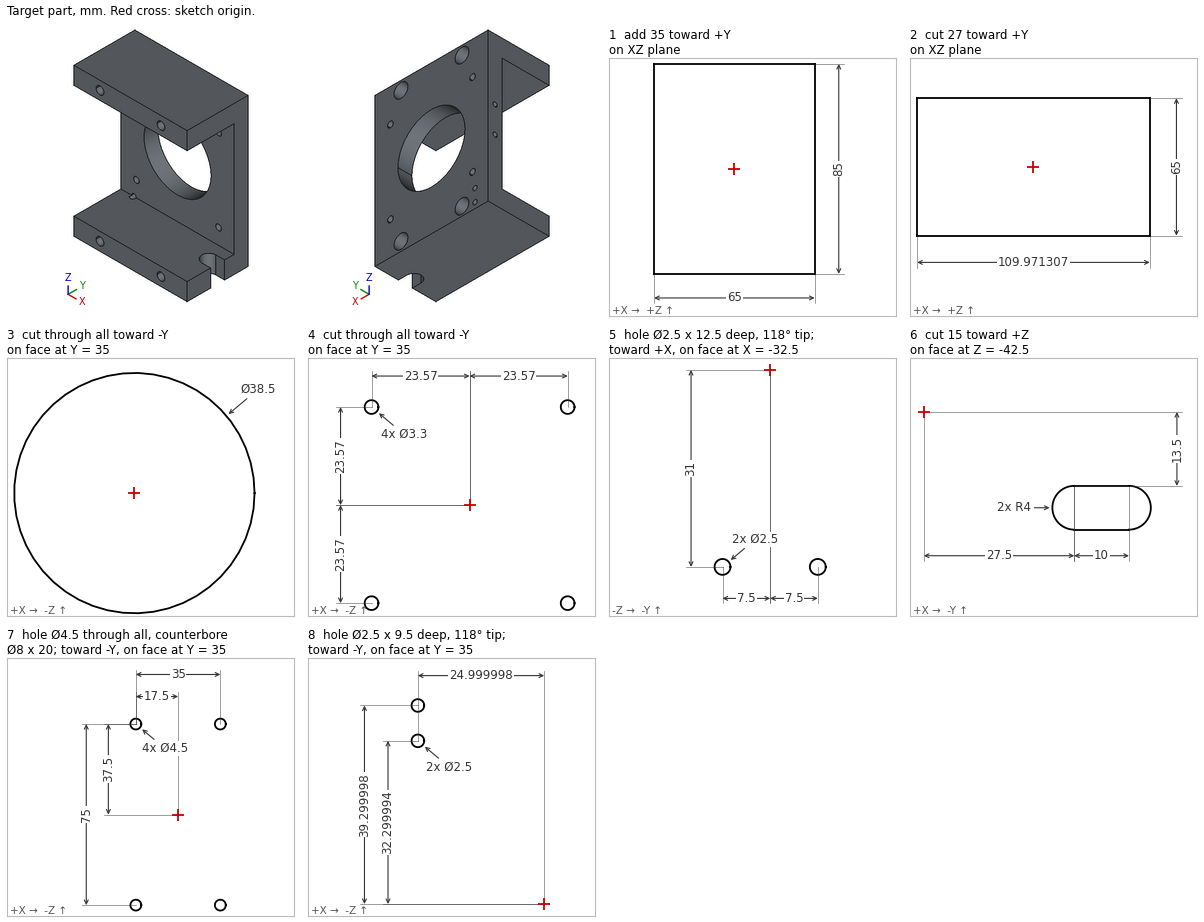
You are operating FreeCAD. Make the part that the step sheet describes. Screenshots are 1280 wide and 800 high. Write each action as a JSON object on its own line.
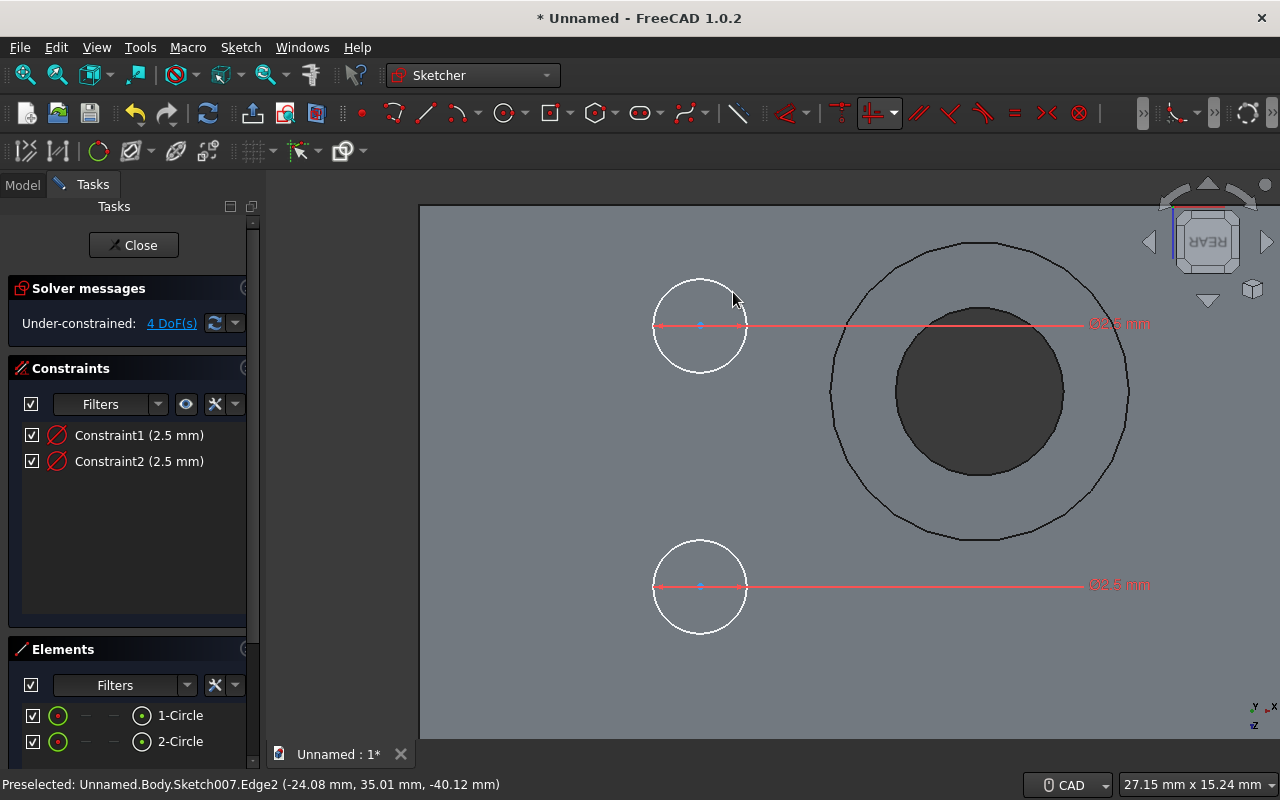
{"action": "left_click", "coordinate": [700, 587]}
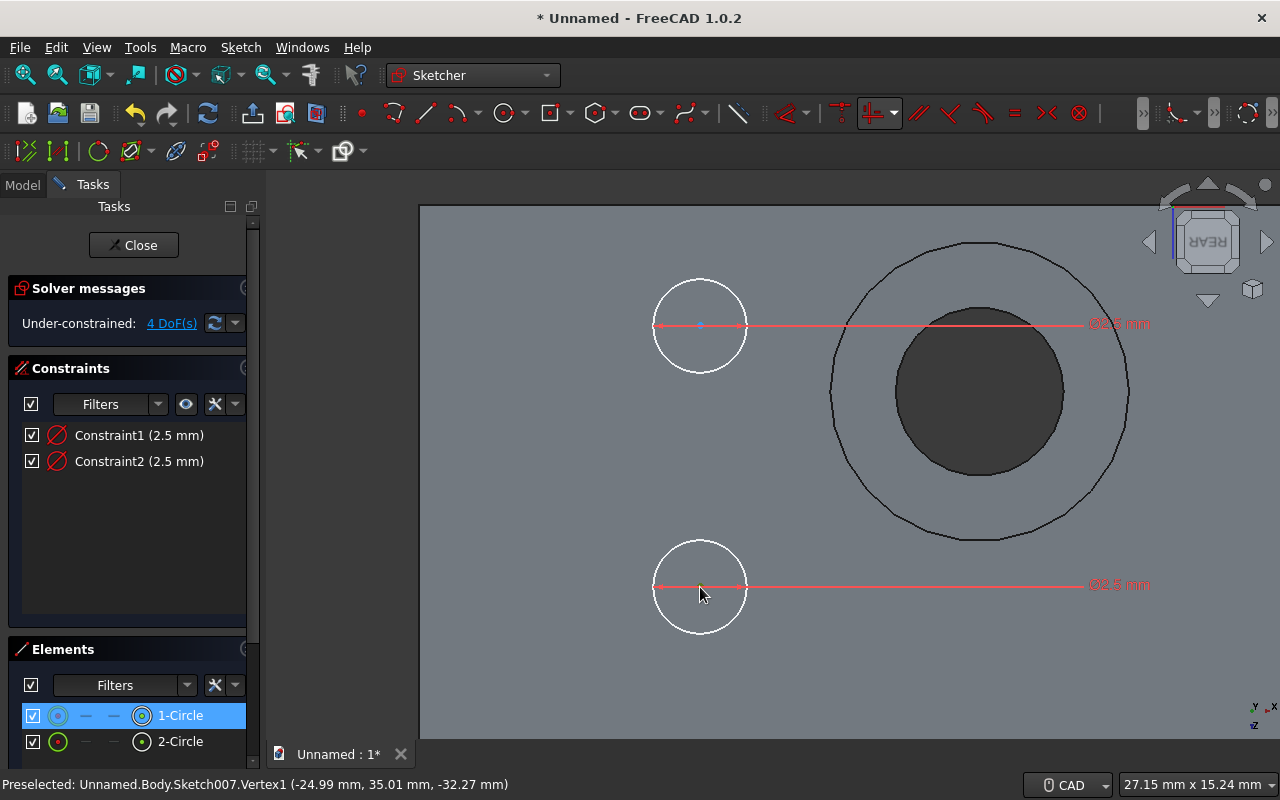
{"action": "left_click", "coordinate": [700, 326]}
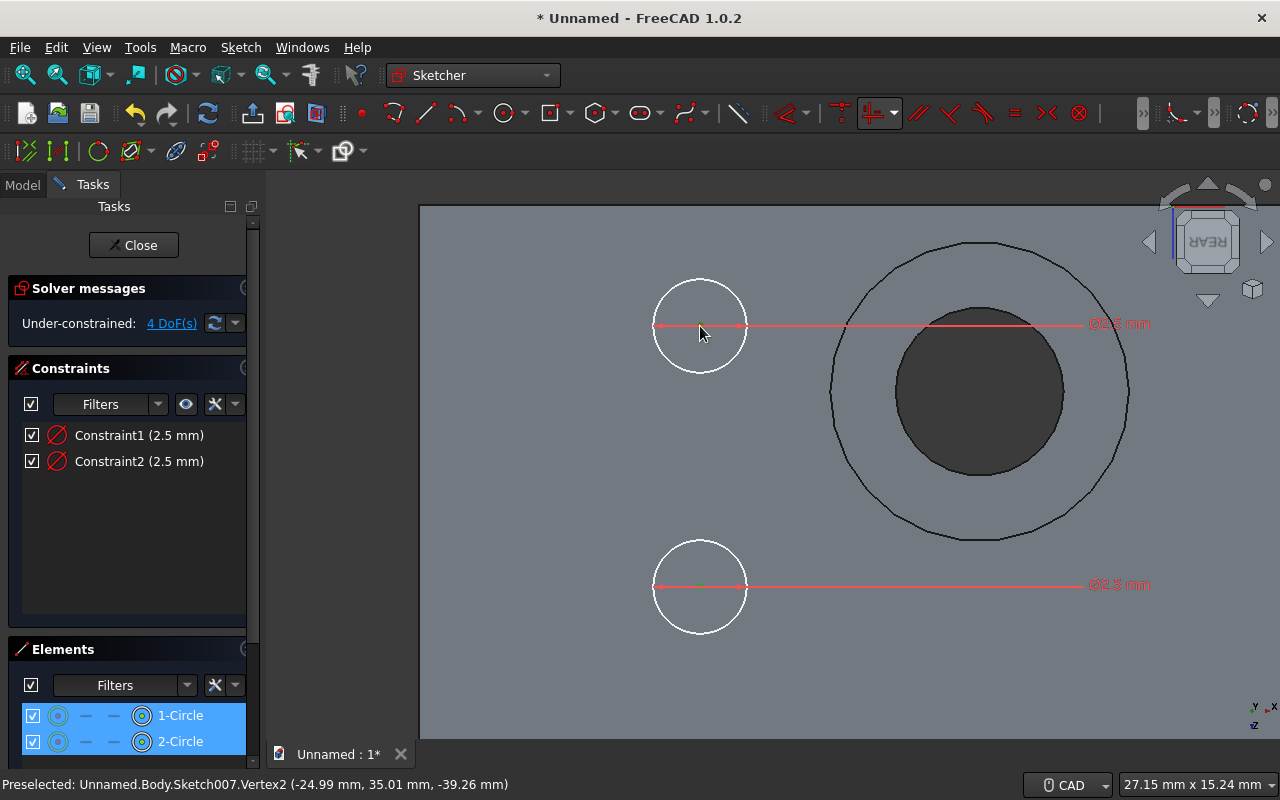
{"action": "key", "text": "v"}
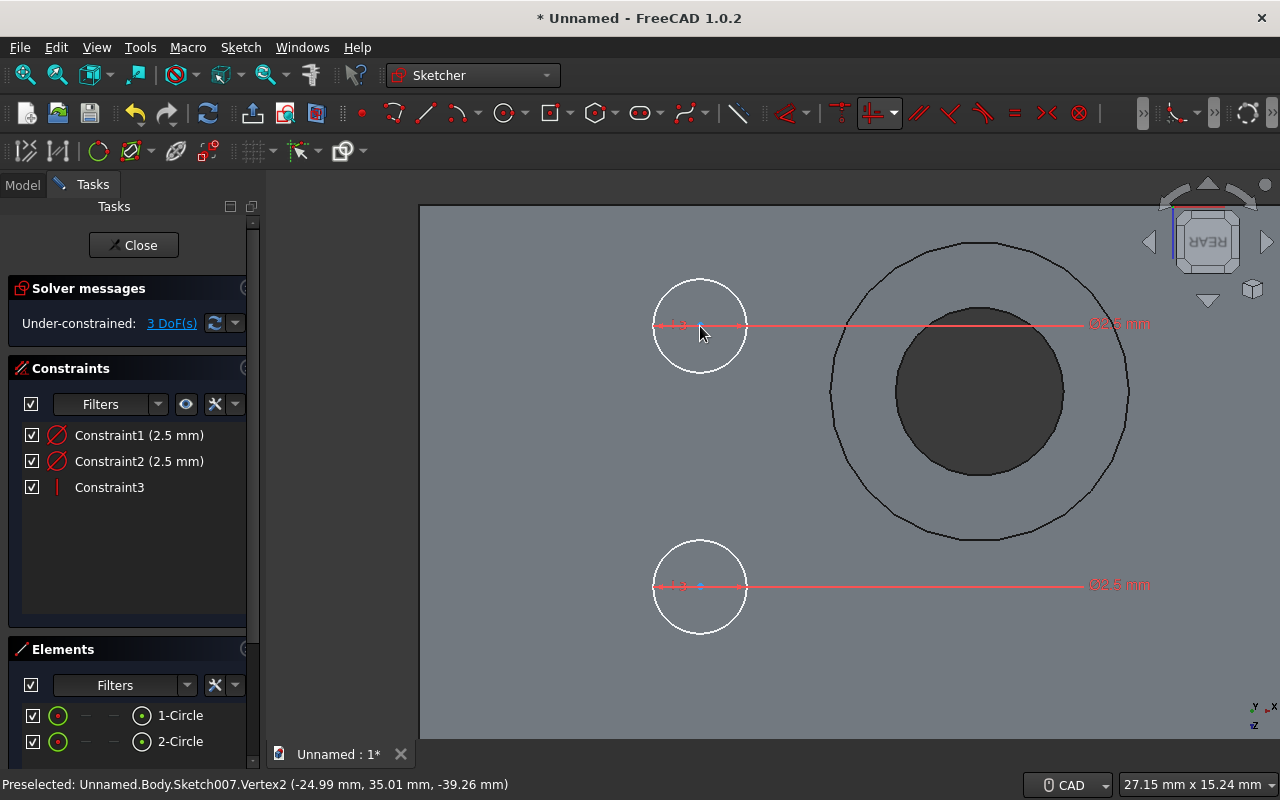
{"action": "left_click", "coordinate": [786, 114]}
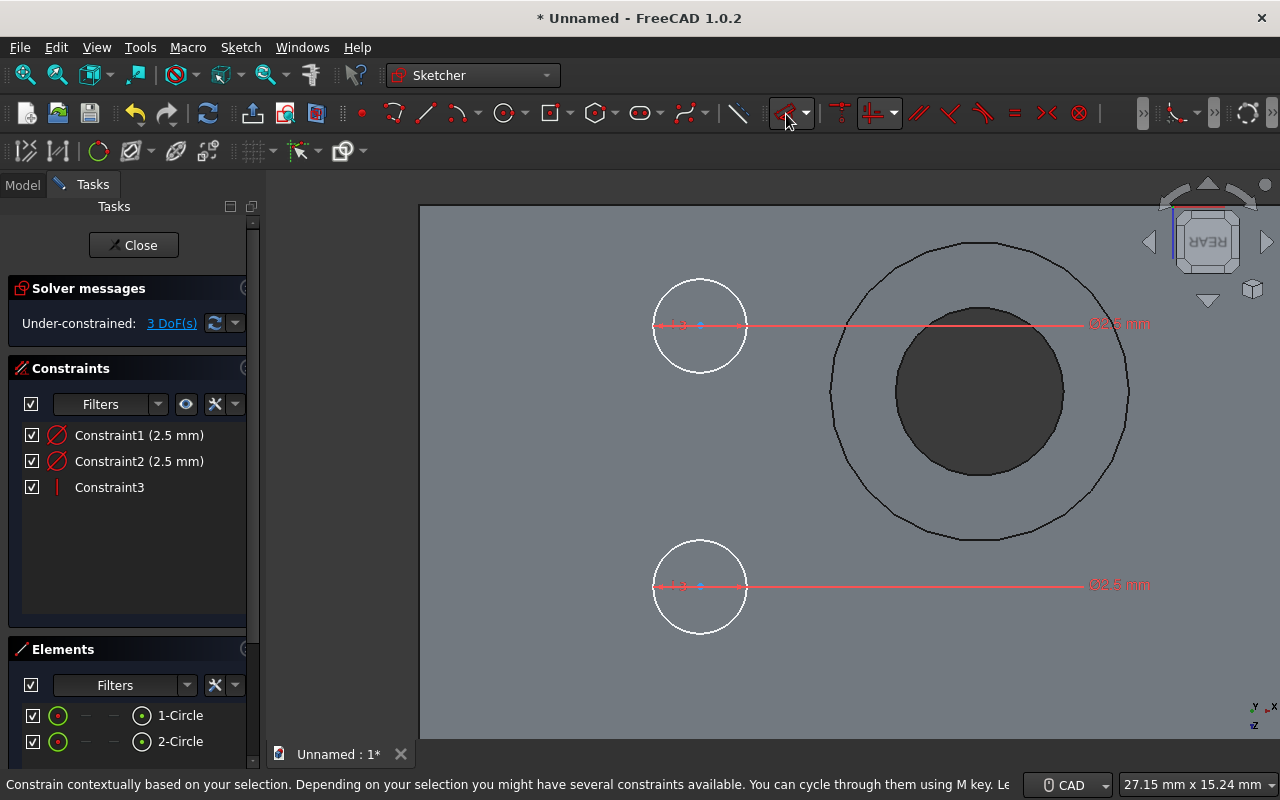
{"action": "left_click", "coordinate": [700, 587]}
{"action": "left_click", "coordinate": [908, 553]}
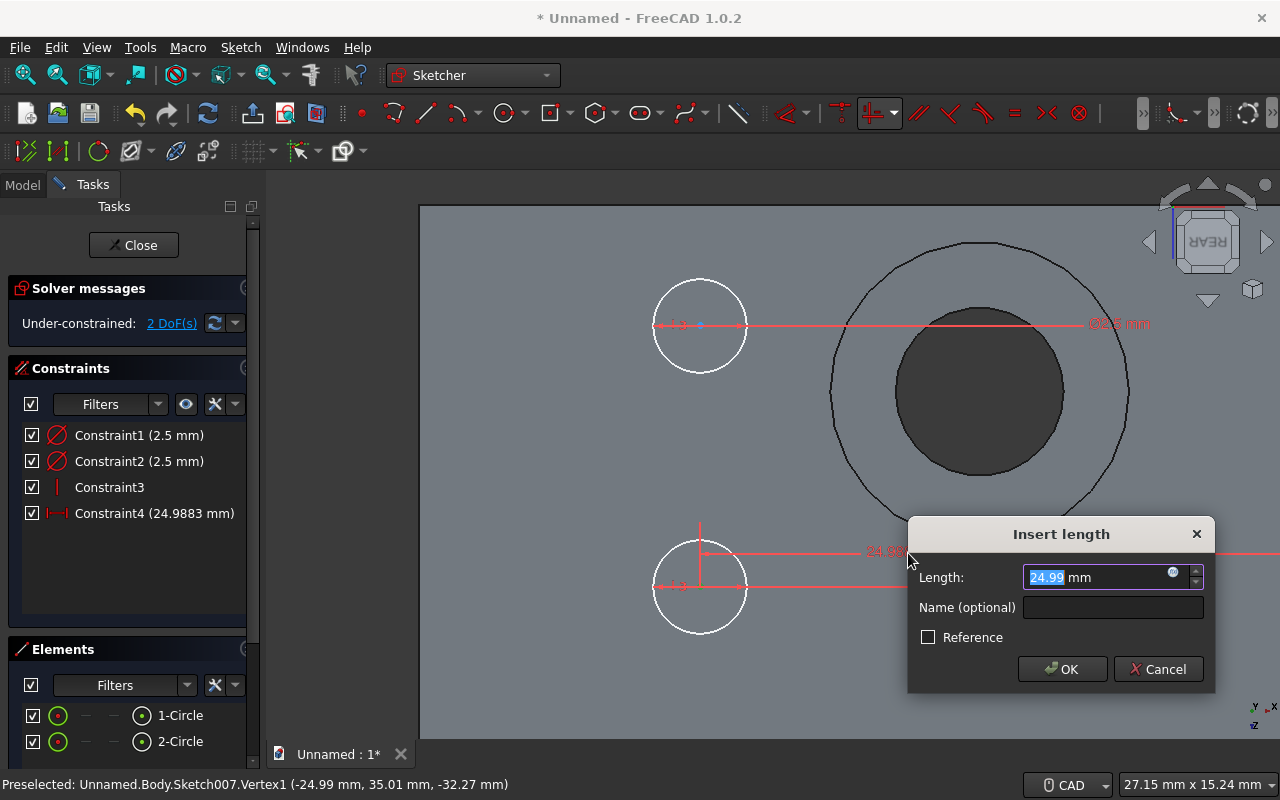
{"action": "type", "text": "24.999998"}
{"action": "key", "text": "Return"}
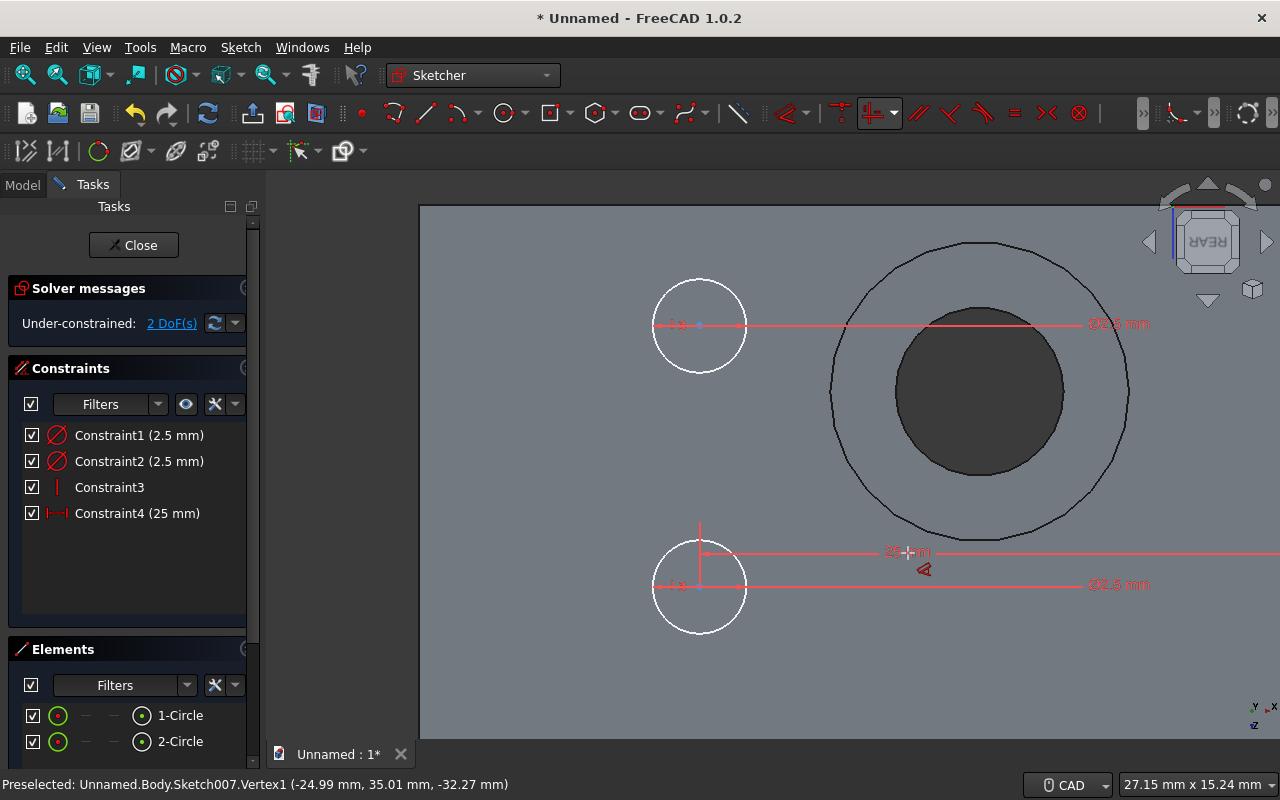
{"action": "left_click", "coordinate": [700, 587]}
{"action": "left_click", "coordinate": [666, 649]}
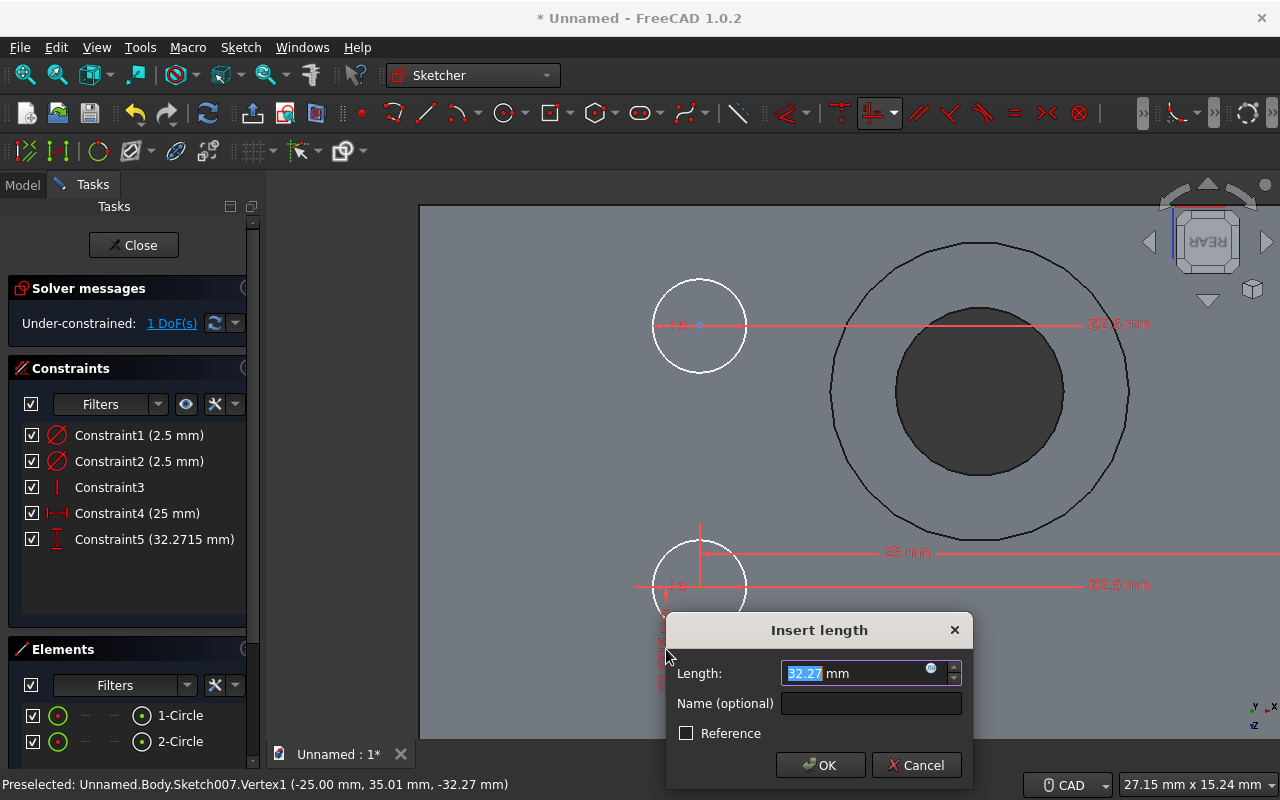
{"action": "type", "text": "32.299994"}
{"action": "key", "text": "Return"}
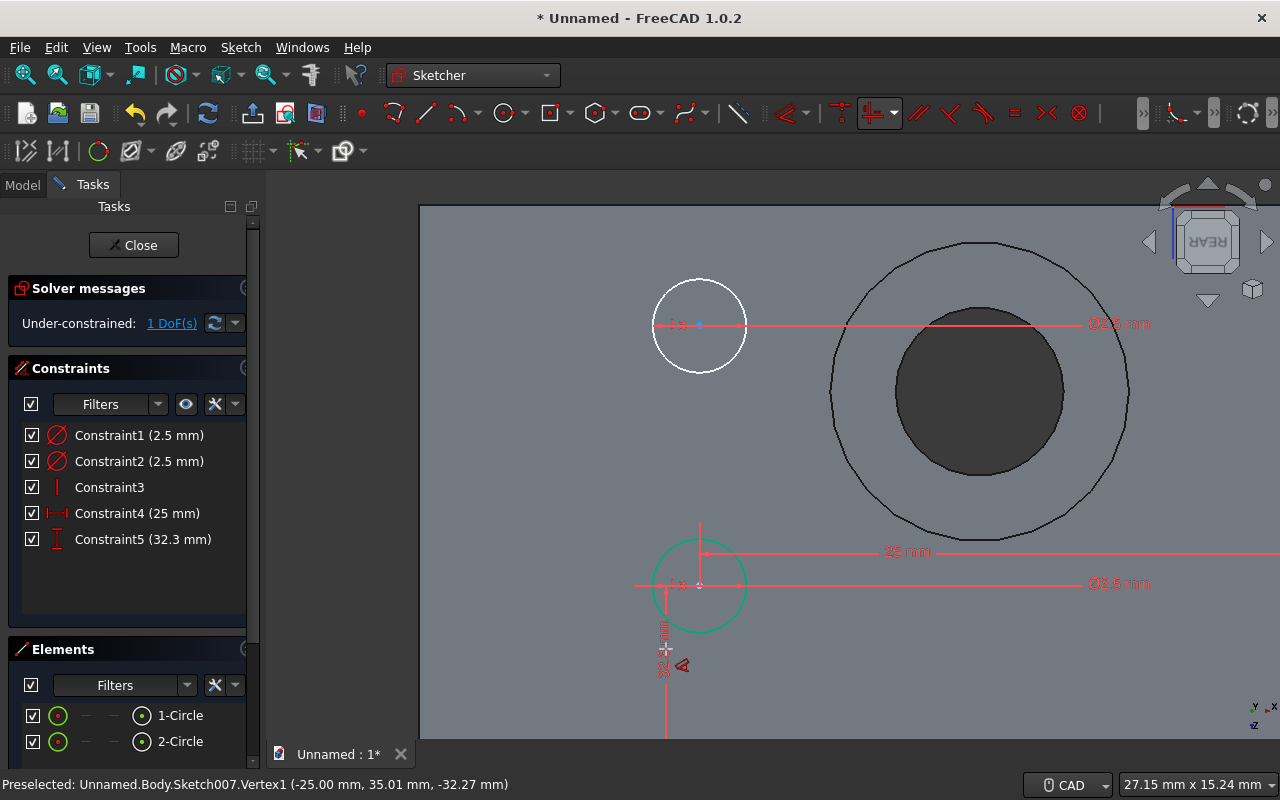
{"action": "left_click", "coordinate": [700, 326]}
{"action": "left_click", "coordinate": [666, 519]}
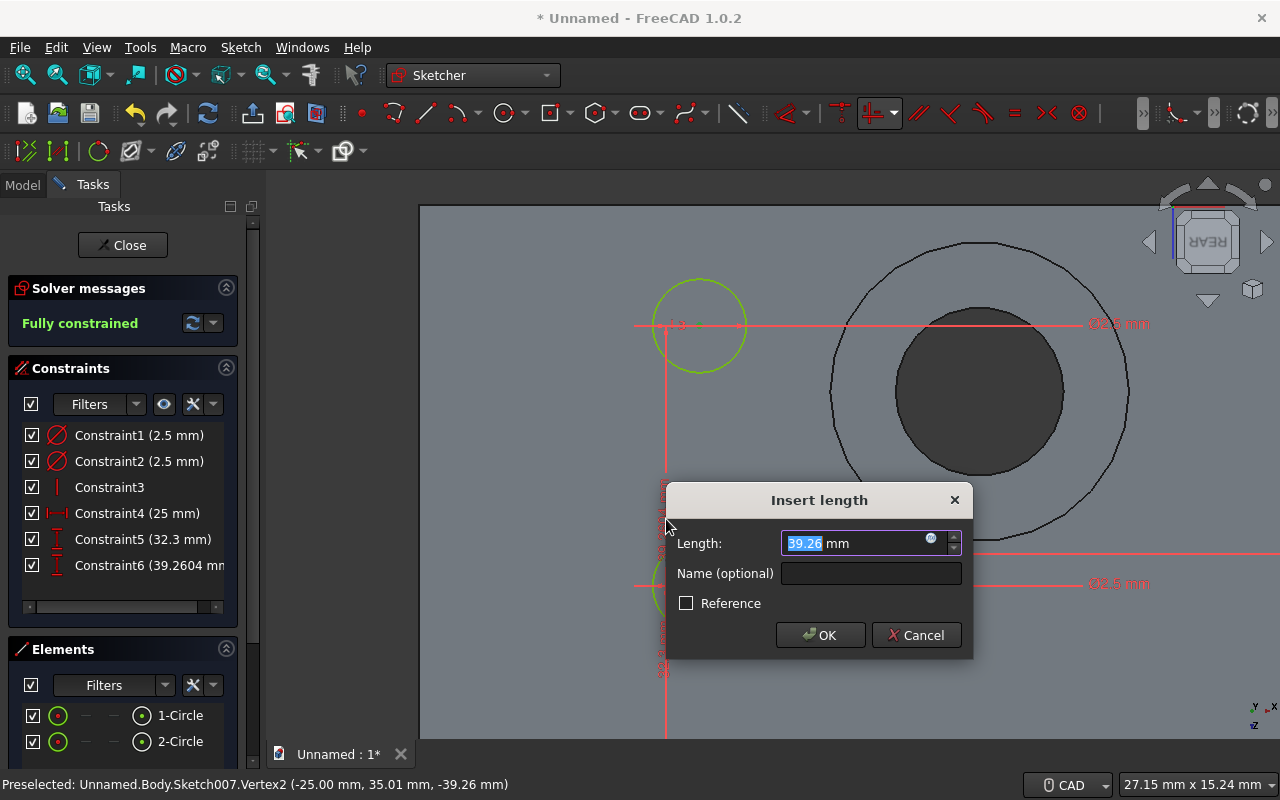
{"action": "type", "text": "39.299998"}
{"action": "key", "text": "Return"}
{"action": "key", "text": "Escape"}